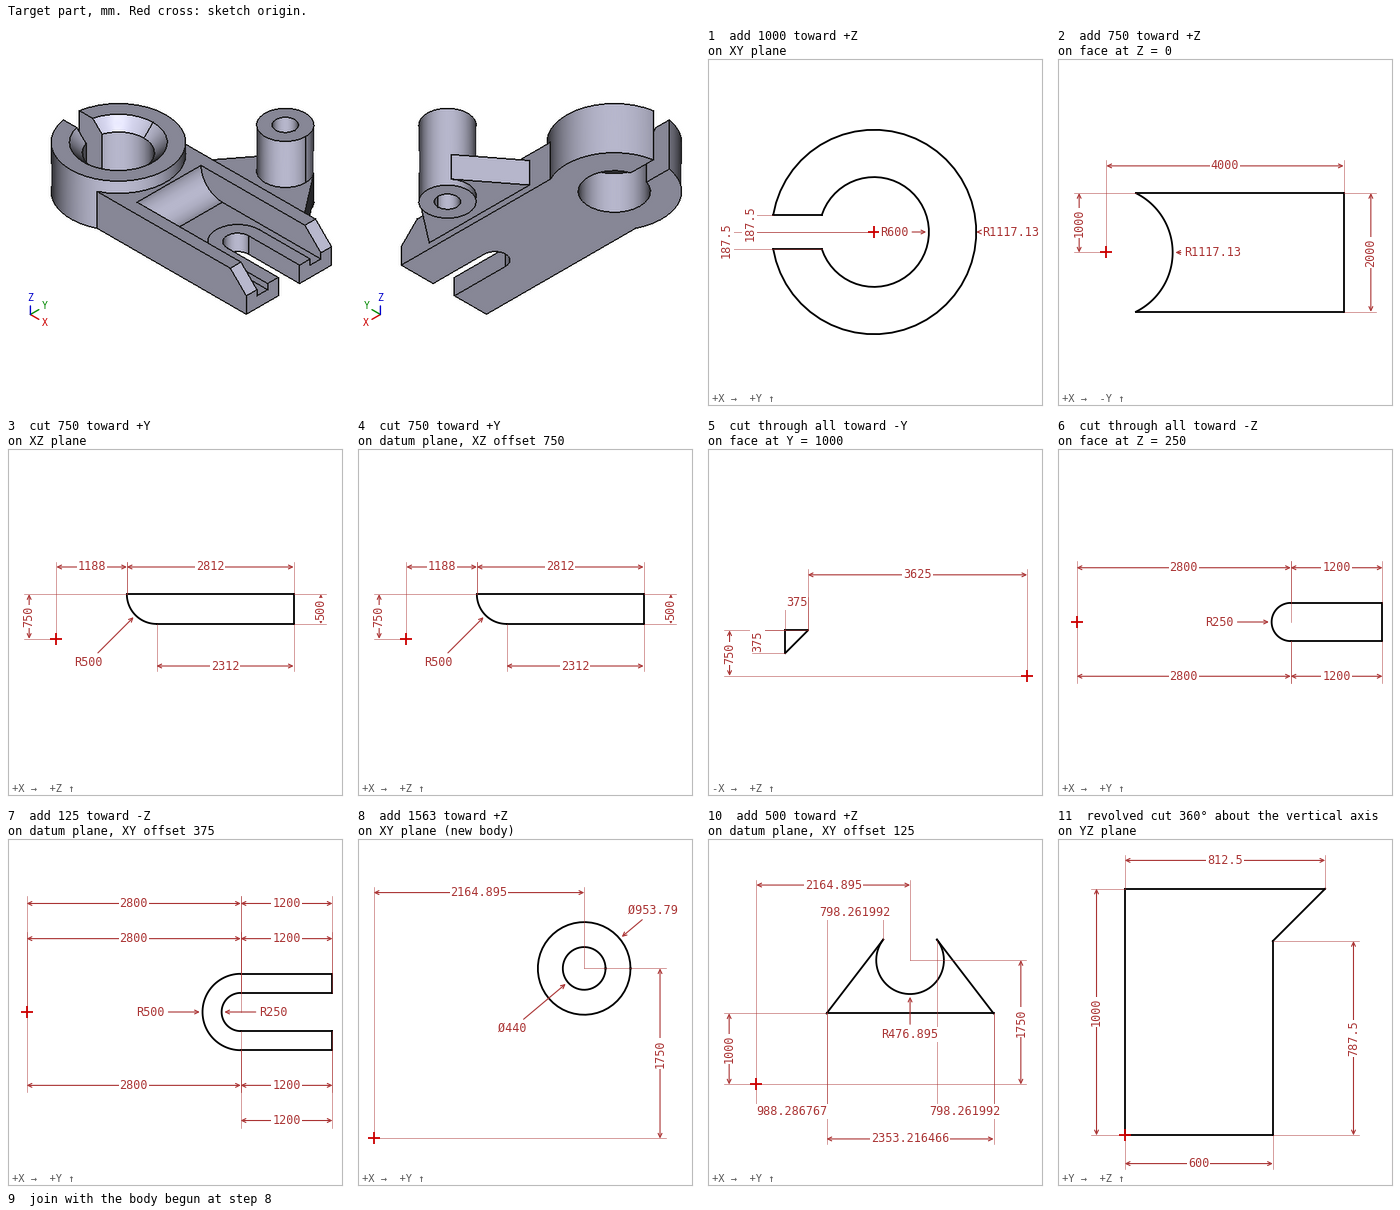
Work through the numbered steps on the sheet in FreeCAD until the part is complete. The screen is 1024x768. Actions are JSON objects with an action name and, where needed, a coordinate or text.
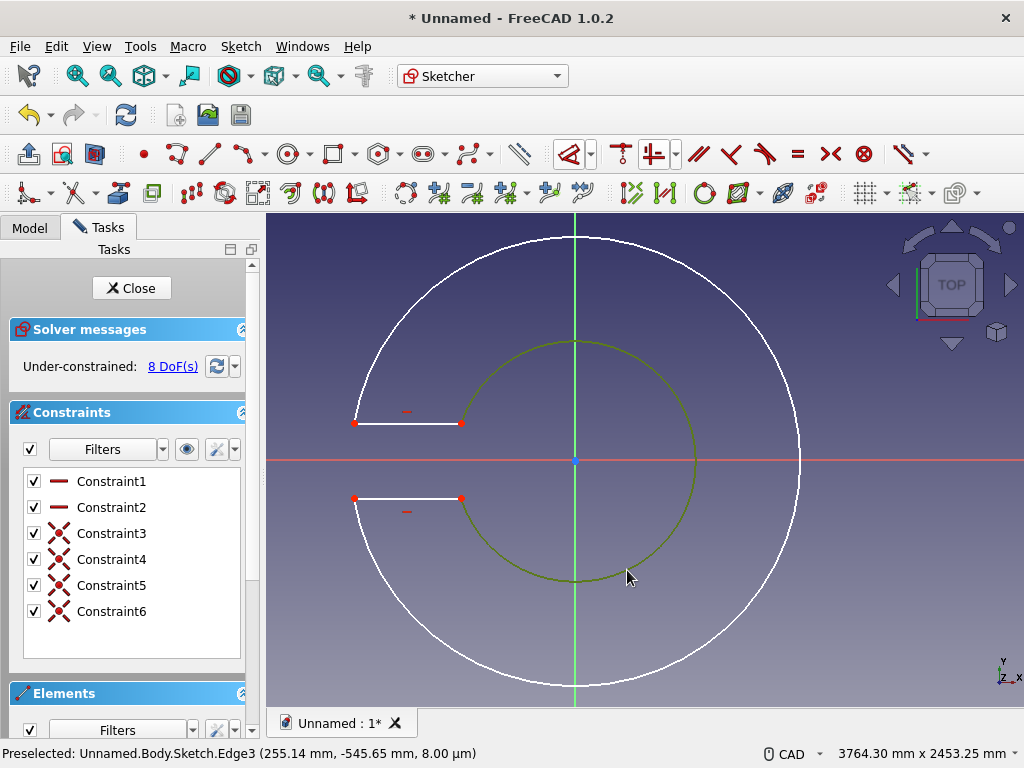
{"action": "left_click", "coordinate": [659, 670]}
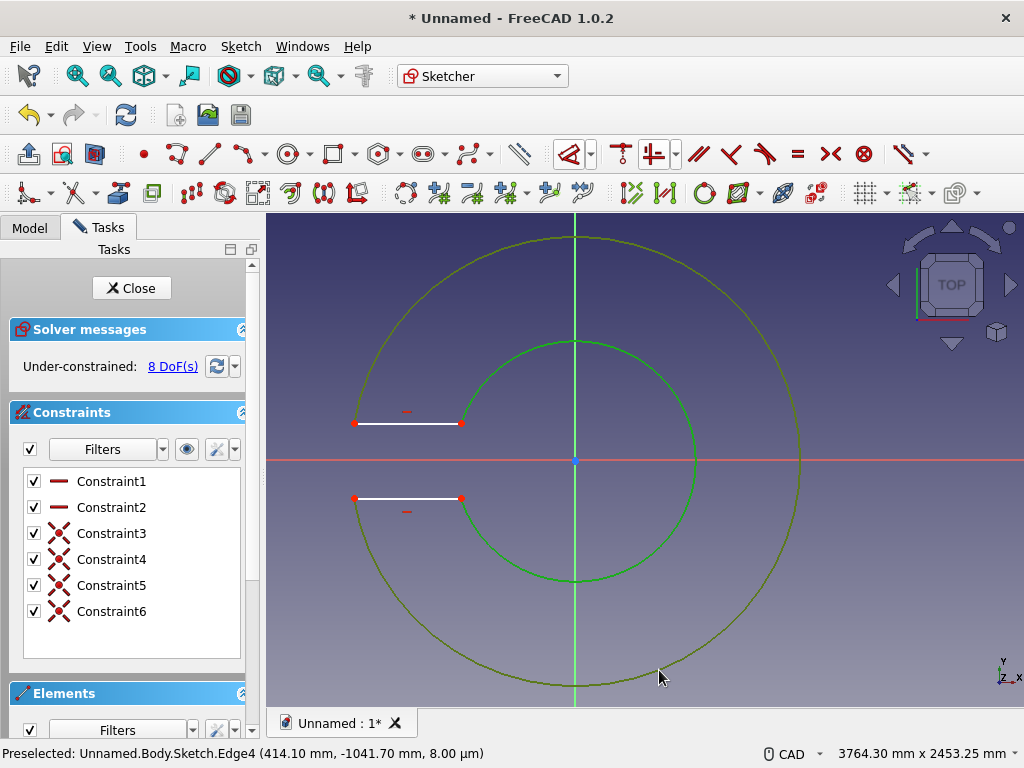
{"action": "left_click", "coordinate": [621, 154]}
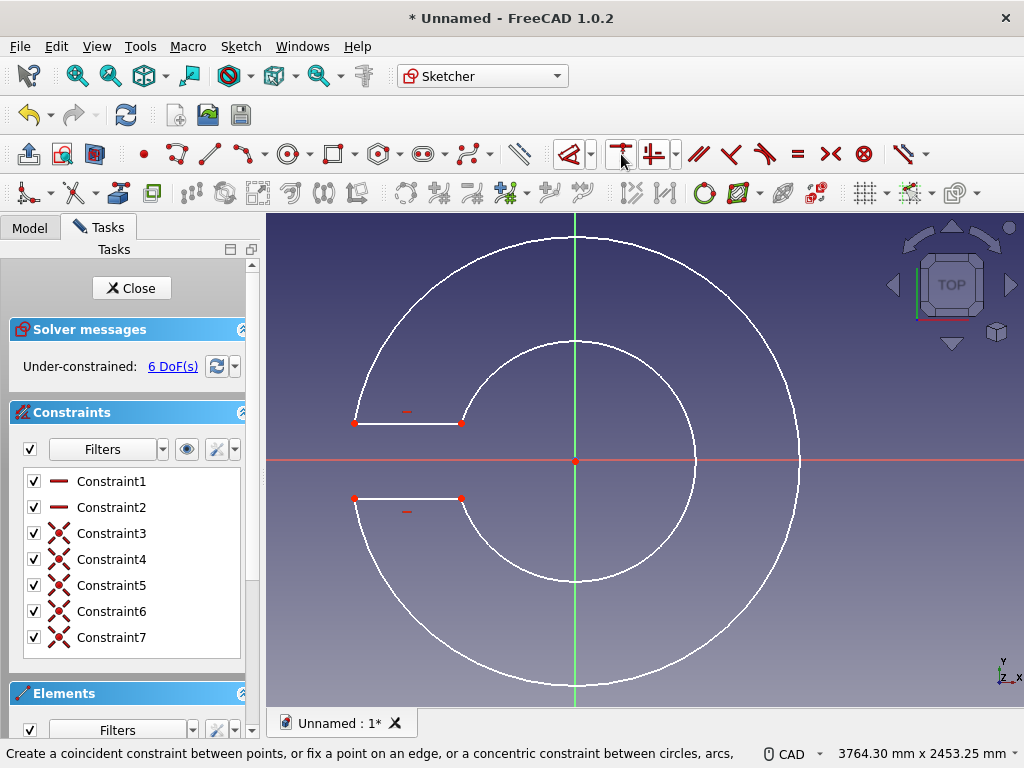
{"action": "left_click_drag", "start_coordinate": [565, 450], "coordinate": [585, 472]}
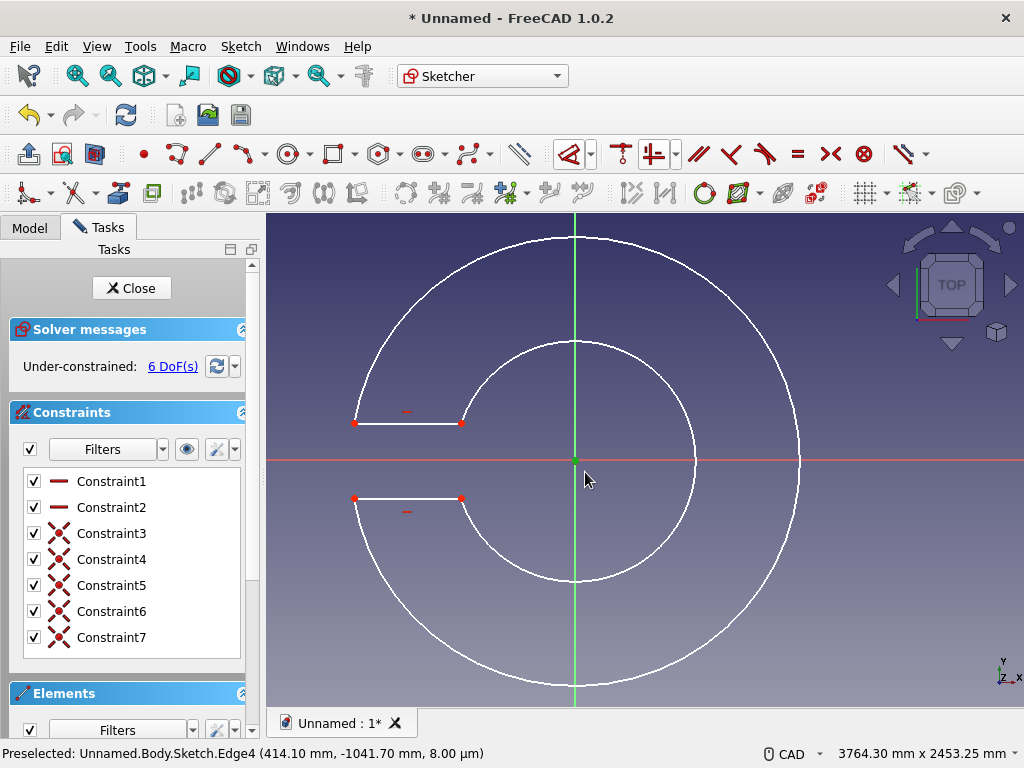
{"action": "key", "text": "c"}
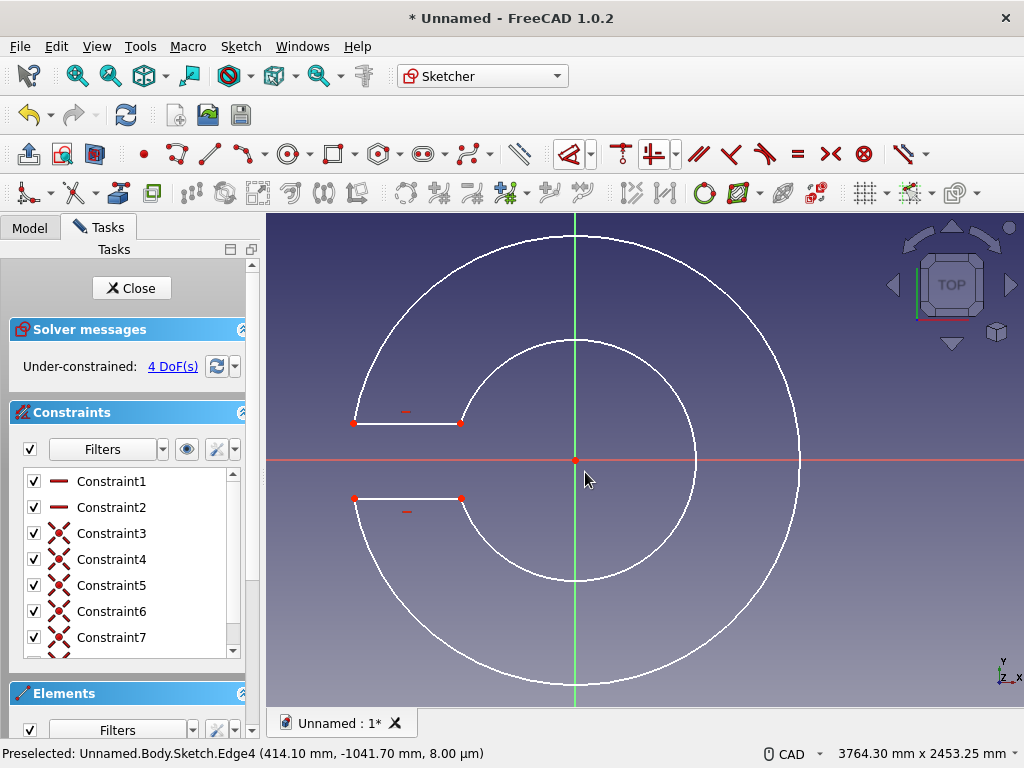
{"action": "key", "text": "d"}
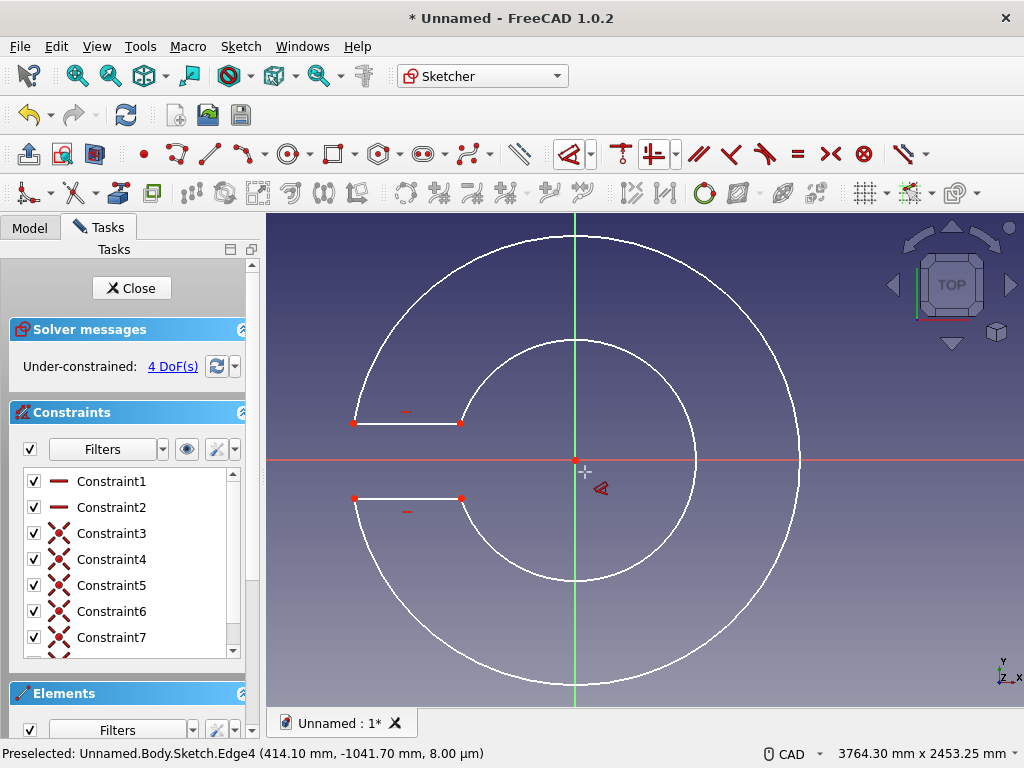
{"action": "left_click", "coordinate": [628, 569]}
{"action": "left_click", "coordinate": [642, 598]}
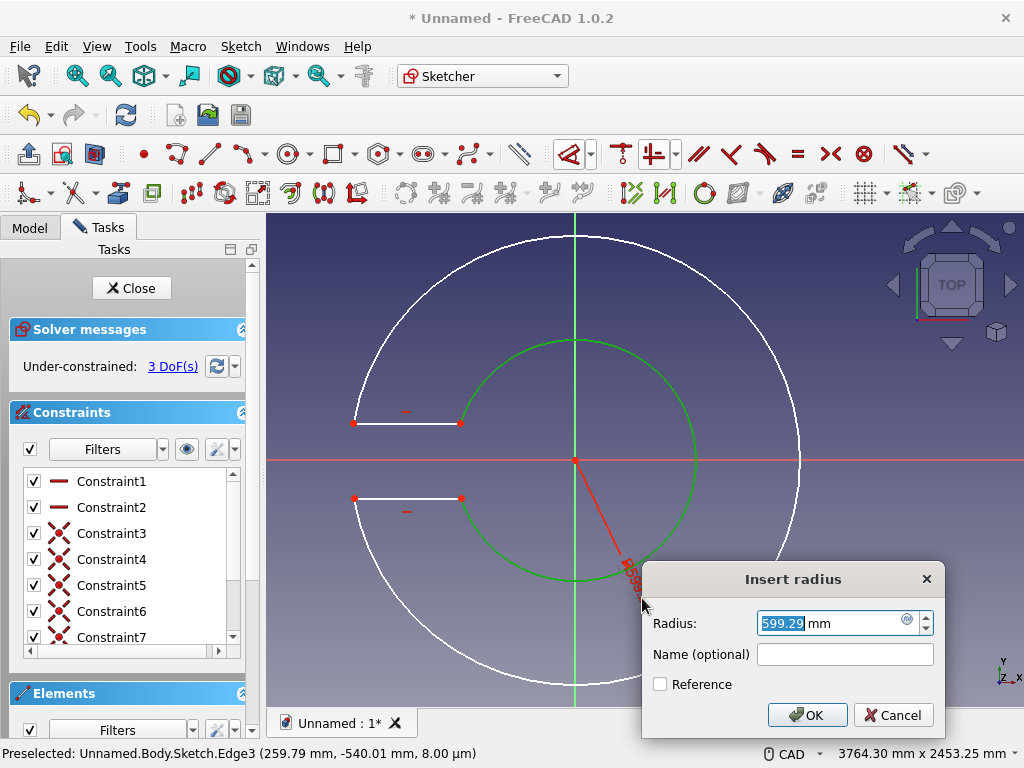
{"action": "type", "text": "600"}
{"action": "key", "text": "Return"}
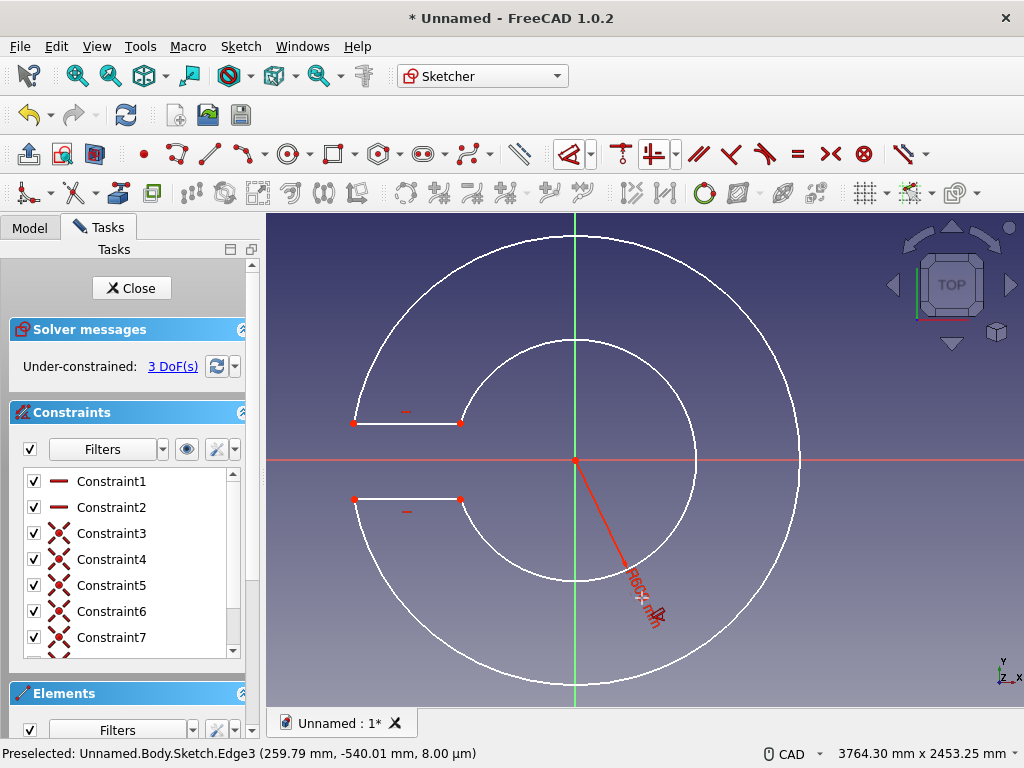
{"action": "left_click", "coordinate": [660, 669]}
{"action": "left_click", "coordinate": [774, 623]}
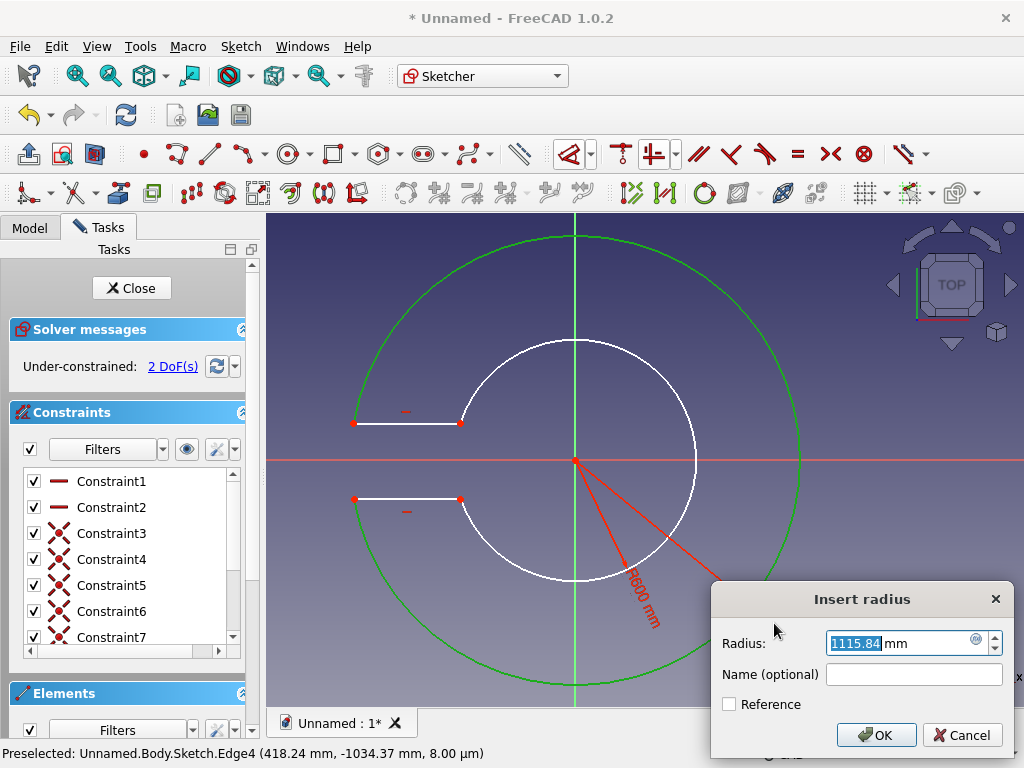
{"action": "type", "text": "1117.13"}
{"action": "key", "text": "Return"}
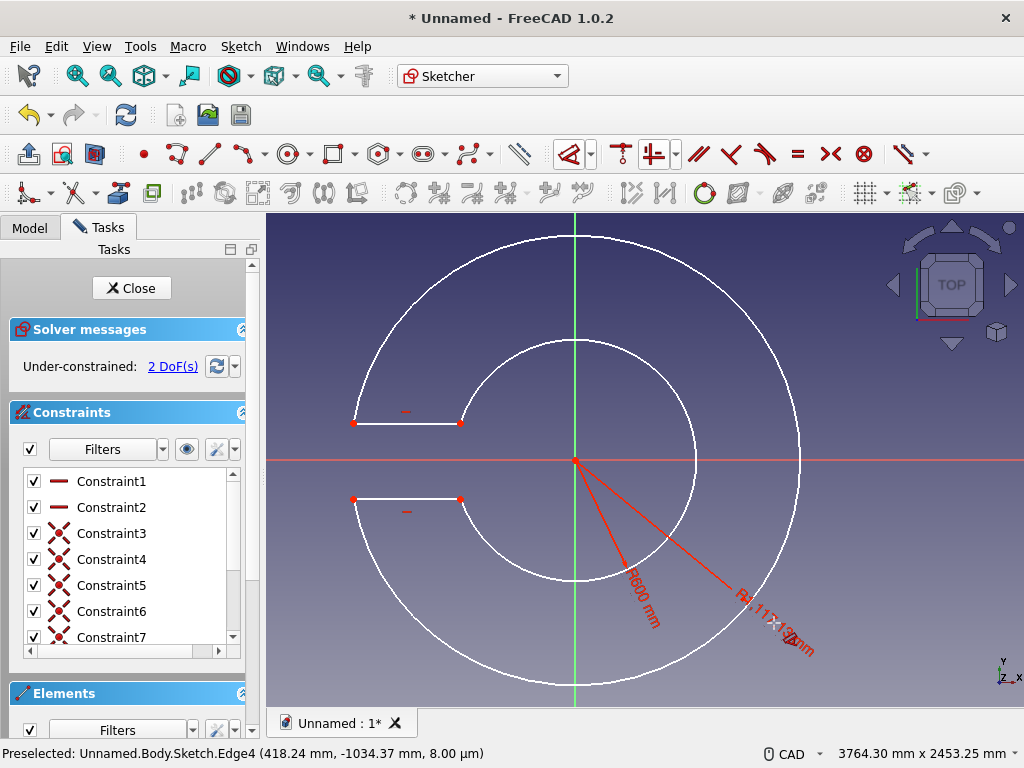
{"action": "left_click", "coordinate": [353, 424]}
{"action": "left_click", "coordinate": [319, 442]}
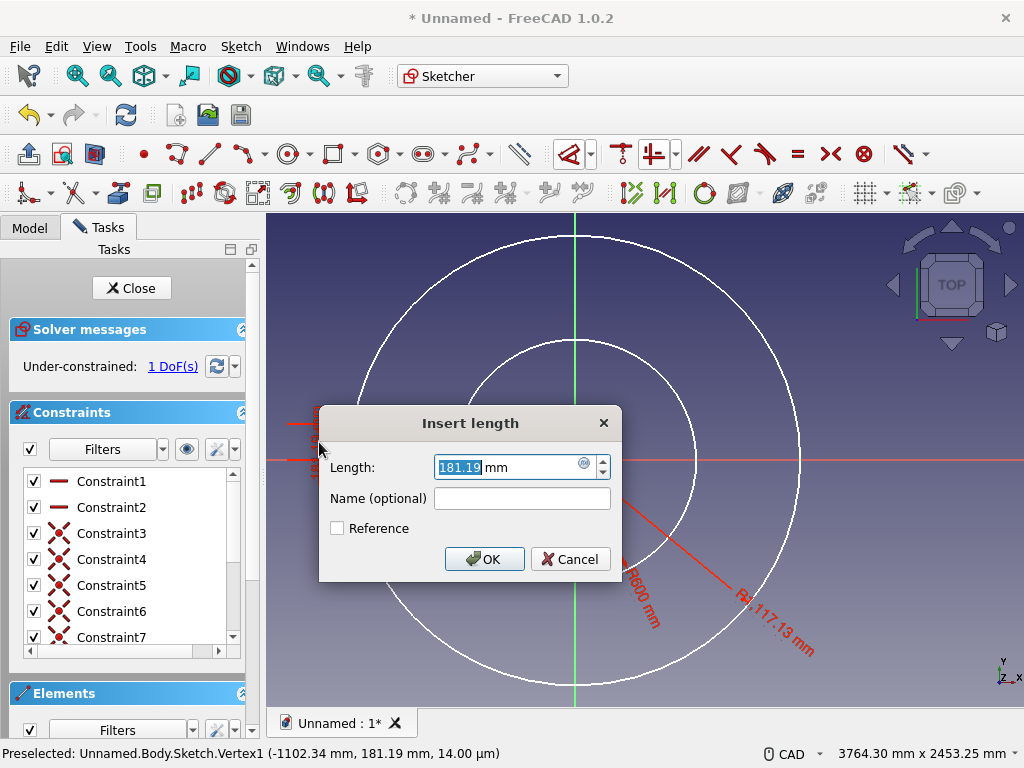
{"action": "type", "text": "187.5"}
{"action": "key", "text": "Return"}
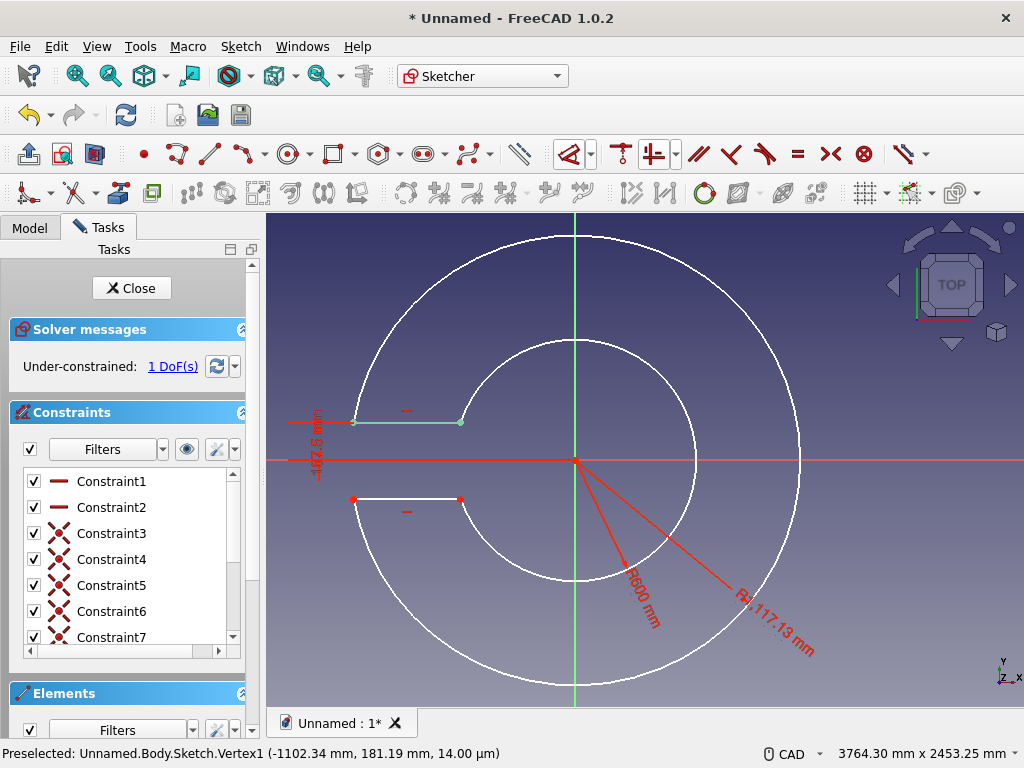
{"action": "left_click", "coordinate": [461, 499]}
{"action": "left_click", "coordinate": [427, 480]}